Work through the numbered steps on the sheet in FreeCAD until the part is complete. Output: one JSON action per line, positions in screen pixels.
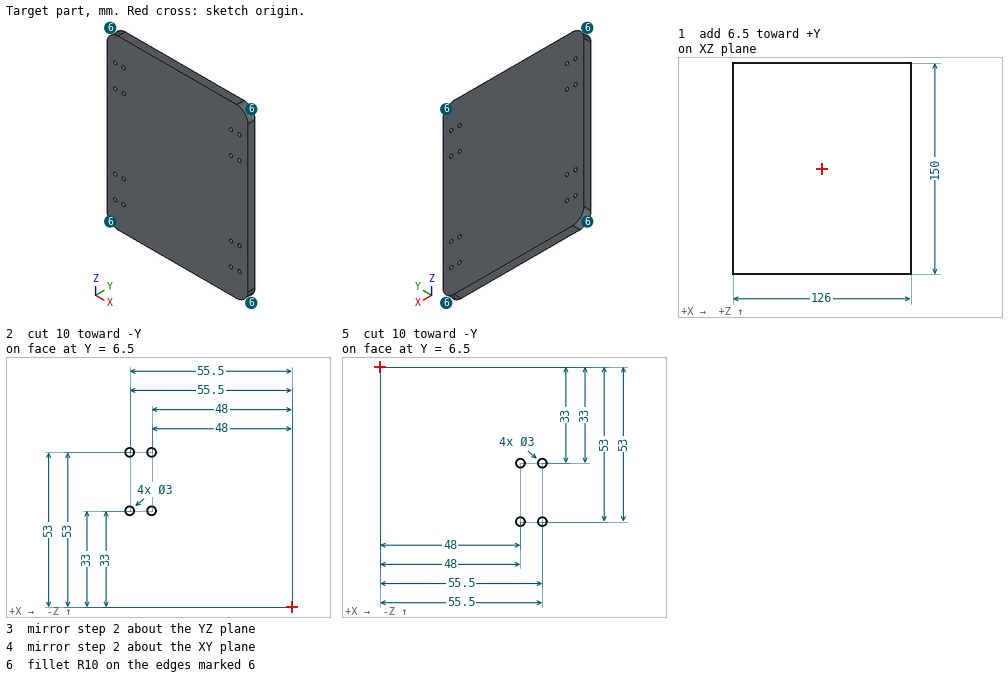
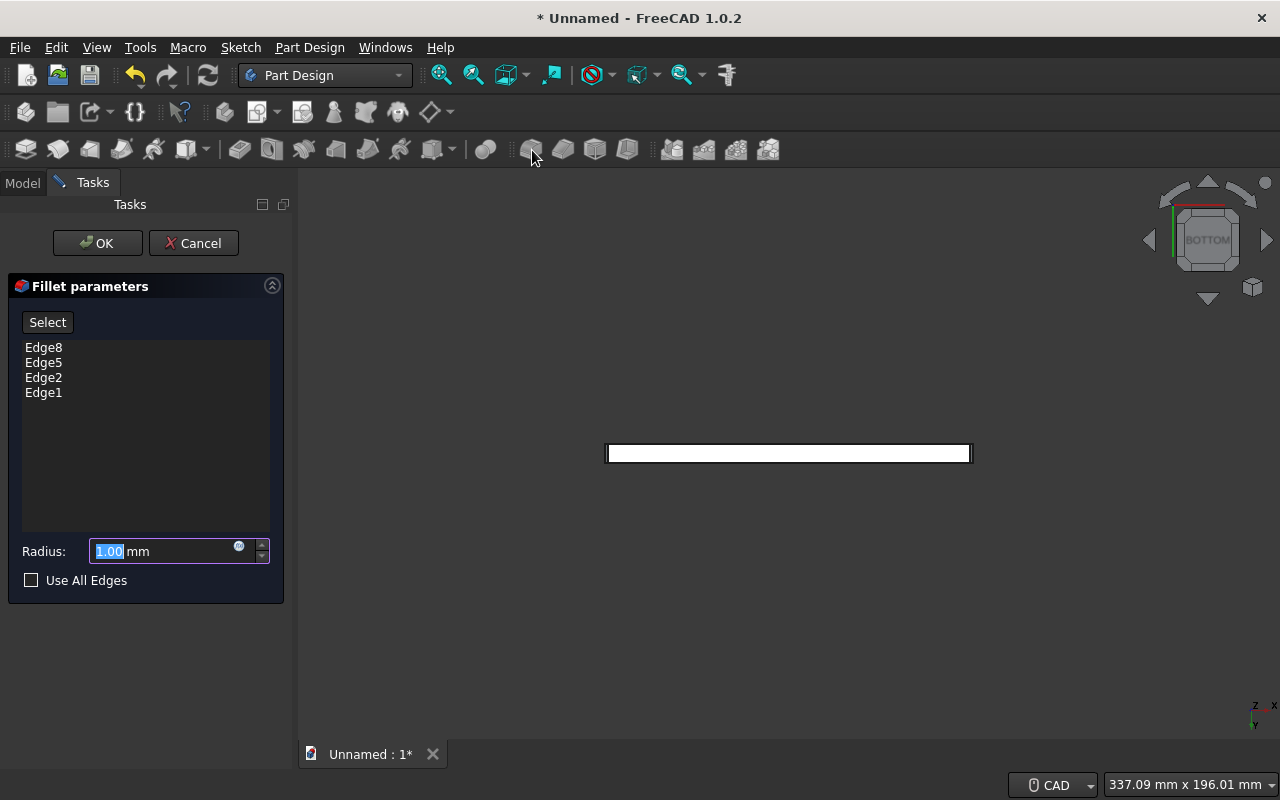
{"action": "type", "text": "10"}
{"action": "key", "text": "Tab"}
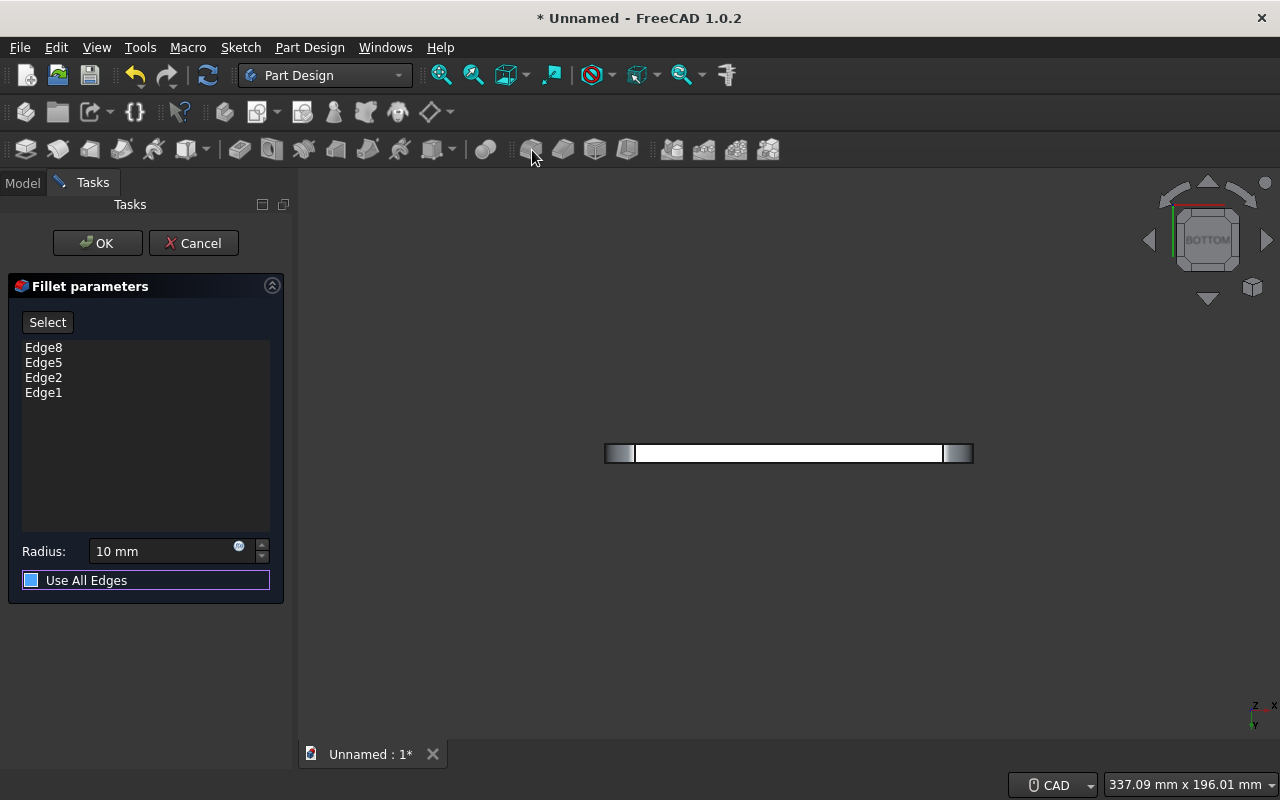
{"action": "left_click", "coordinate": [98, 243]}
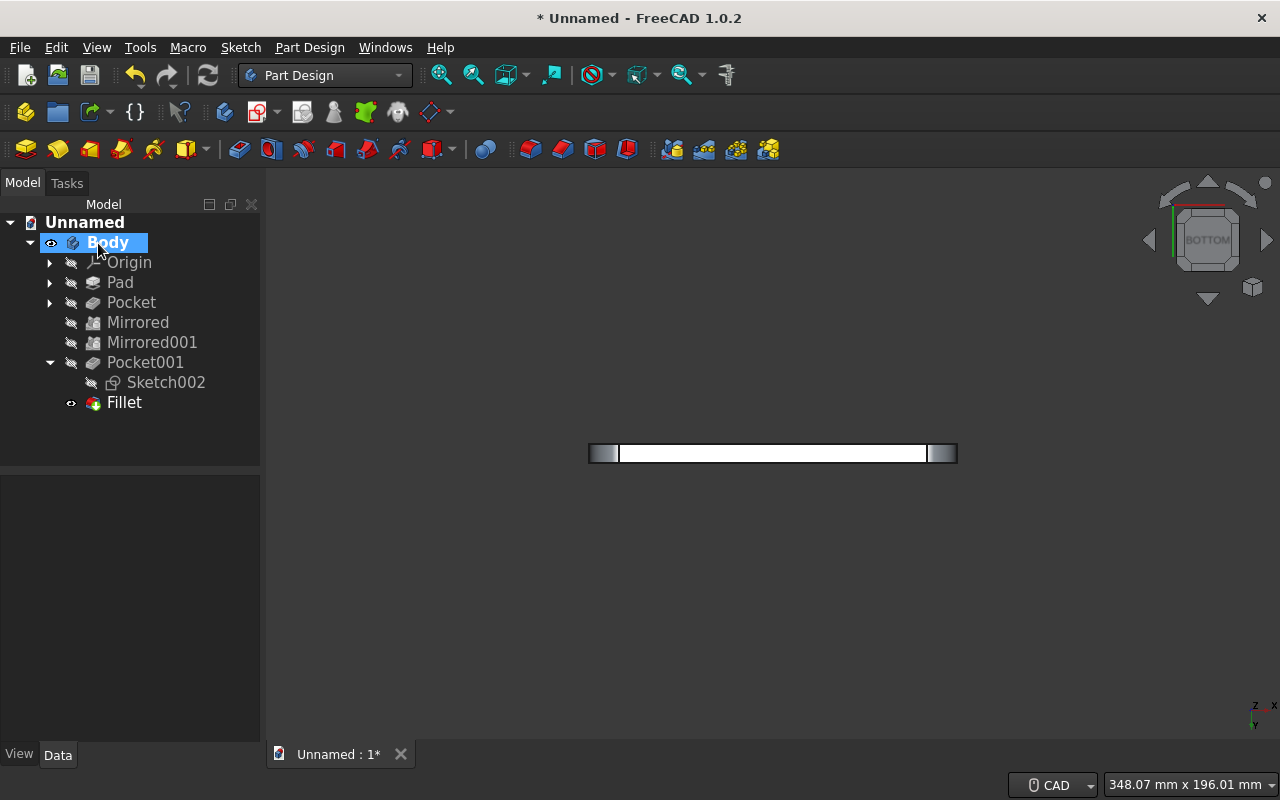
{"action": "key", "text": "0"}